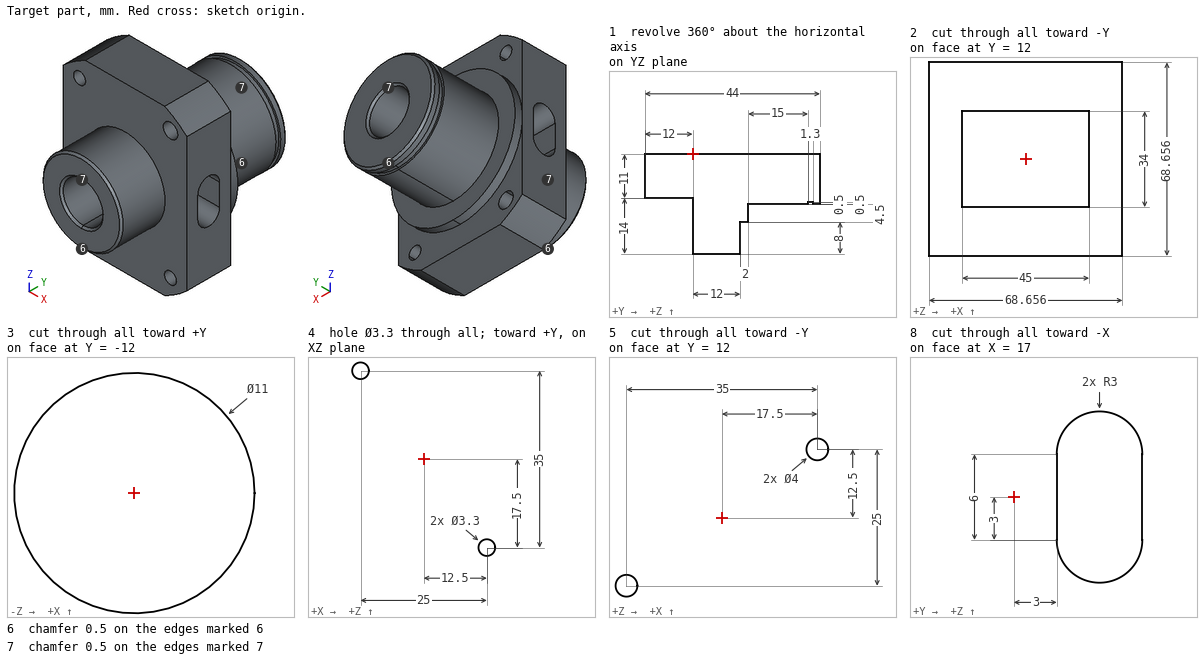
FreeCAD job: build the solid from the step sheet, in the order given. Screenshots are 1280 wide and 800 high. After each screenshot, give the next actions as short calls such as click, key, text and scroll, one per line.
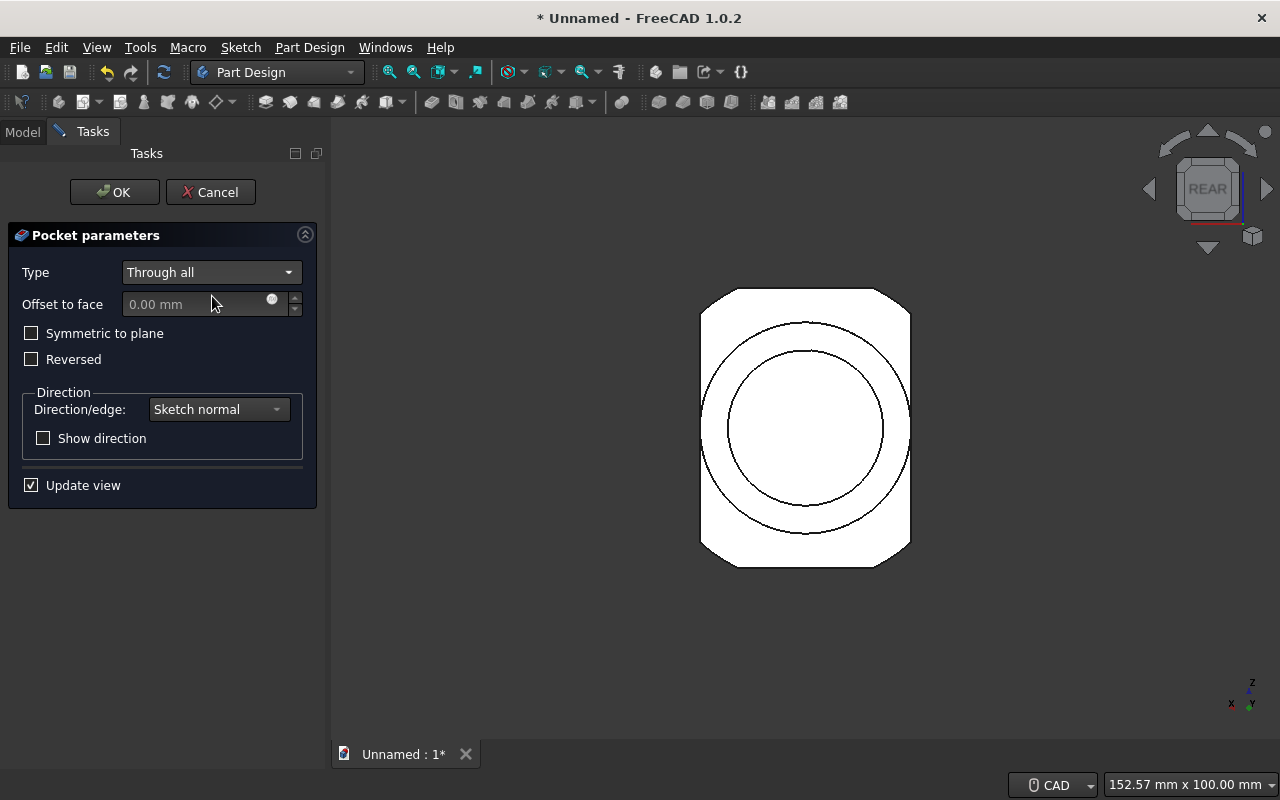
click(115, 192)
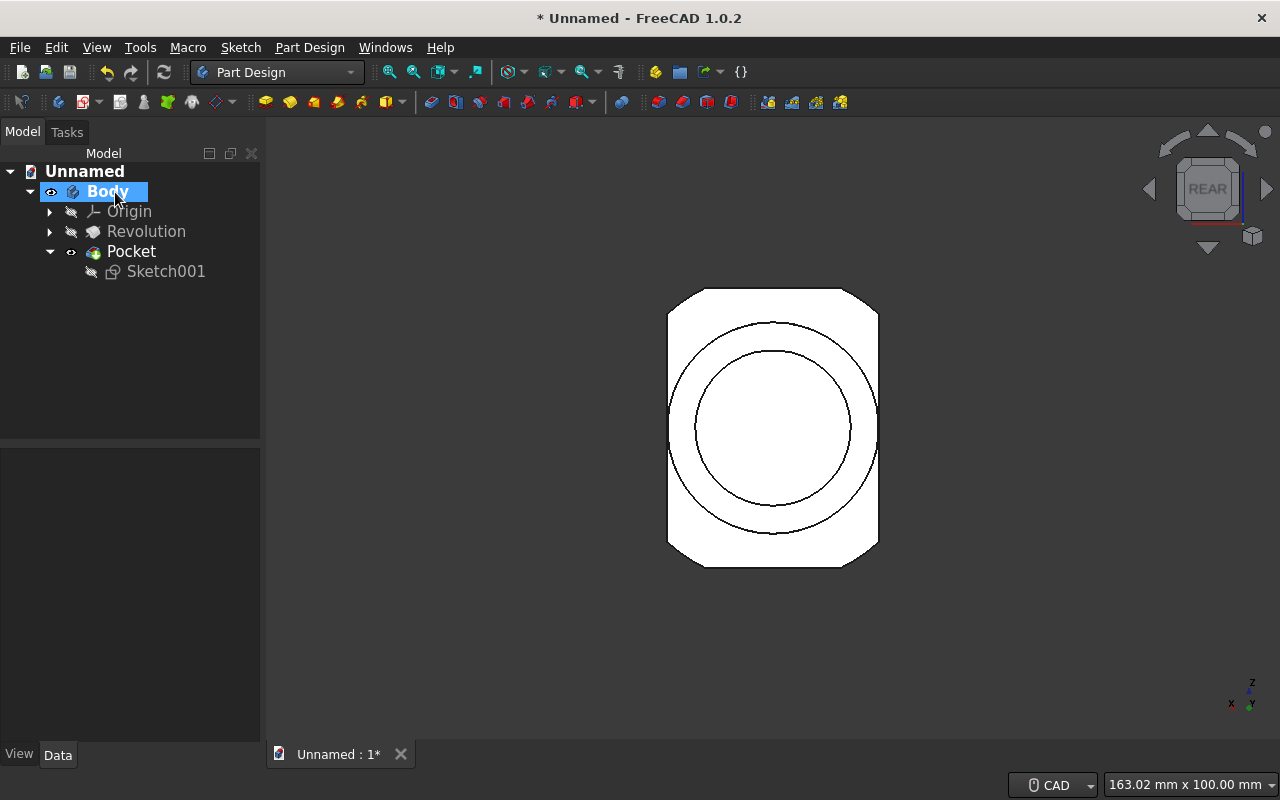
key(0)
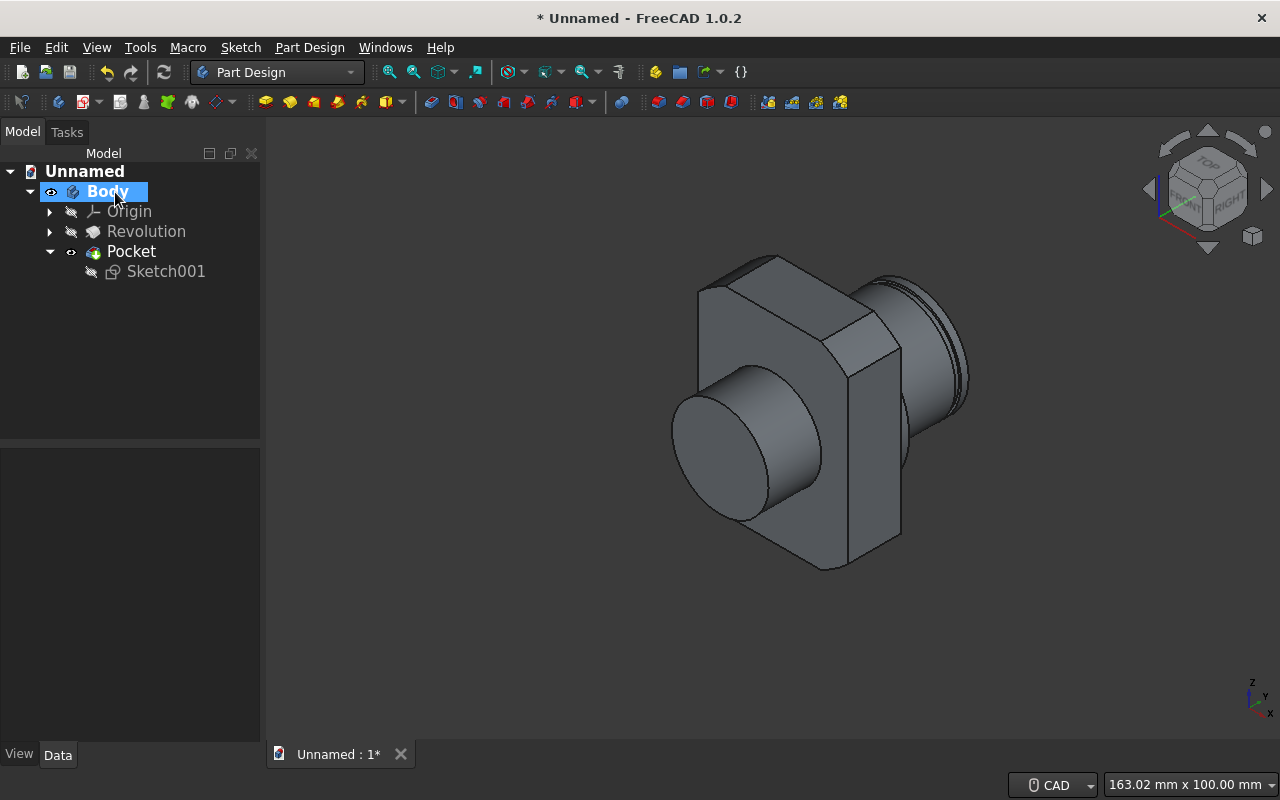
click(720, 457)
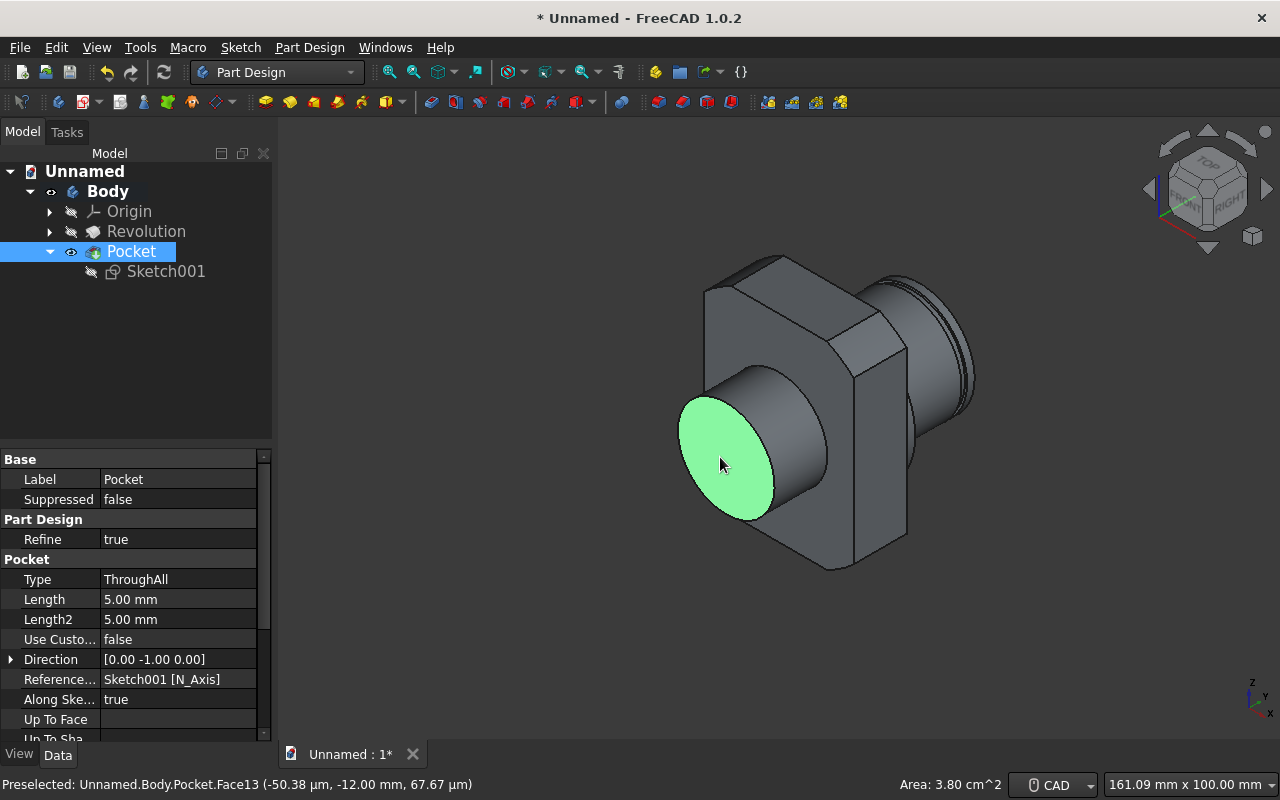
click(84, 102)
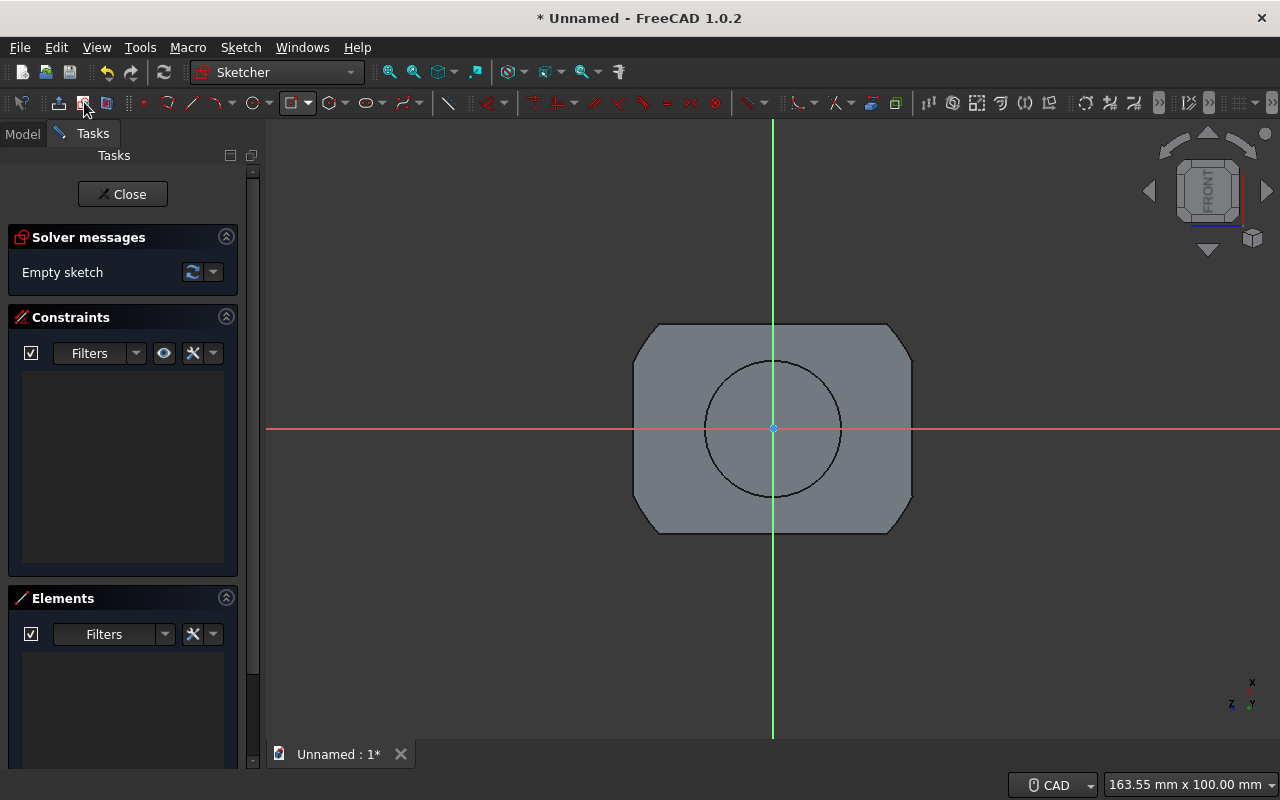
scroll(787, 429, up, 9)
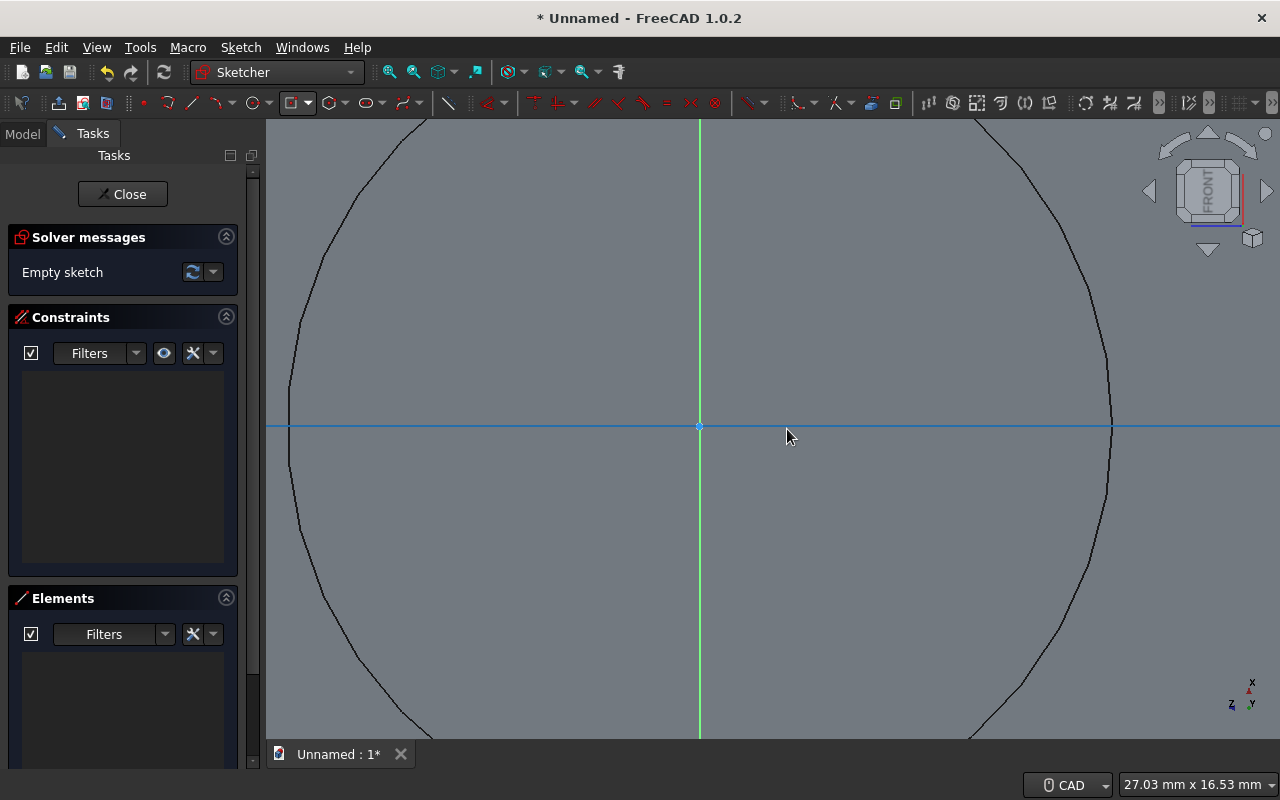
click(254, 104)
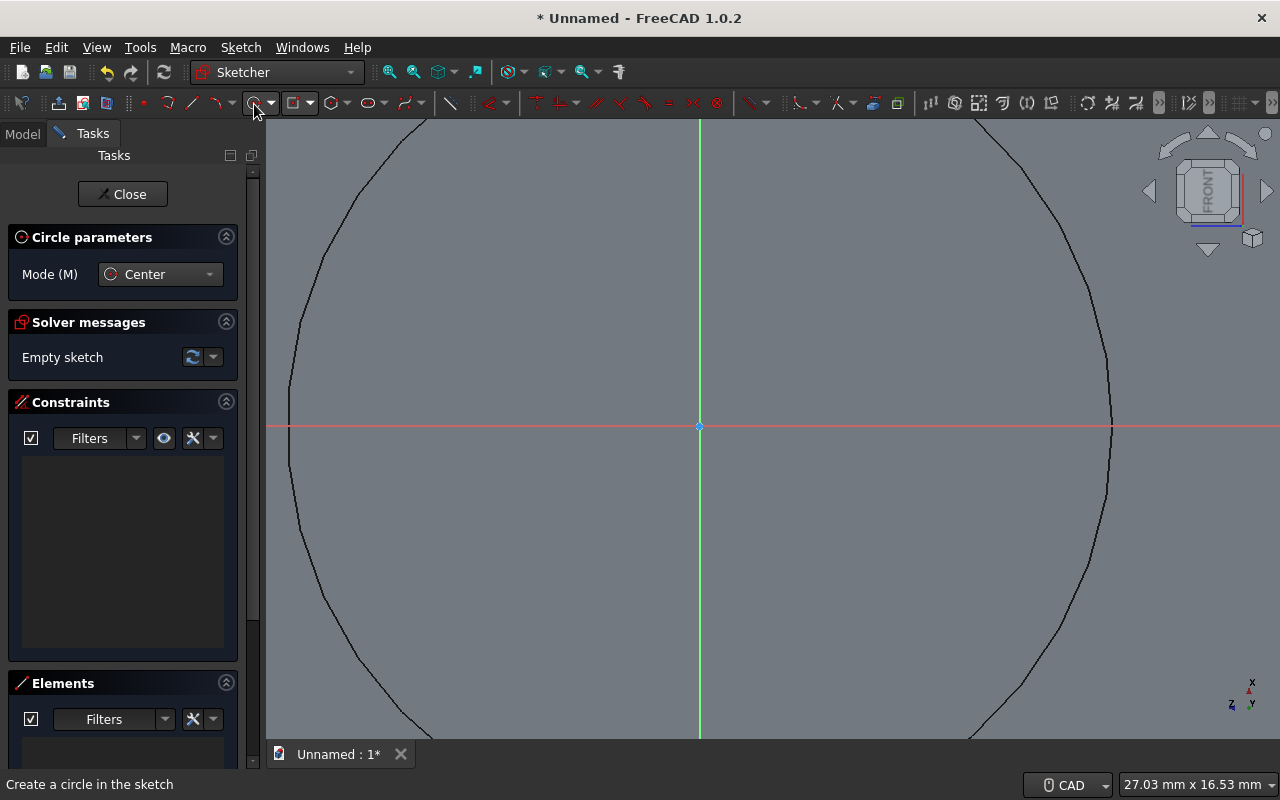
click(700, 426)
move(846, 281)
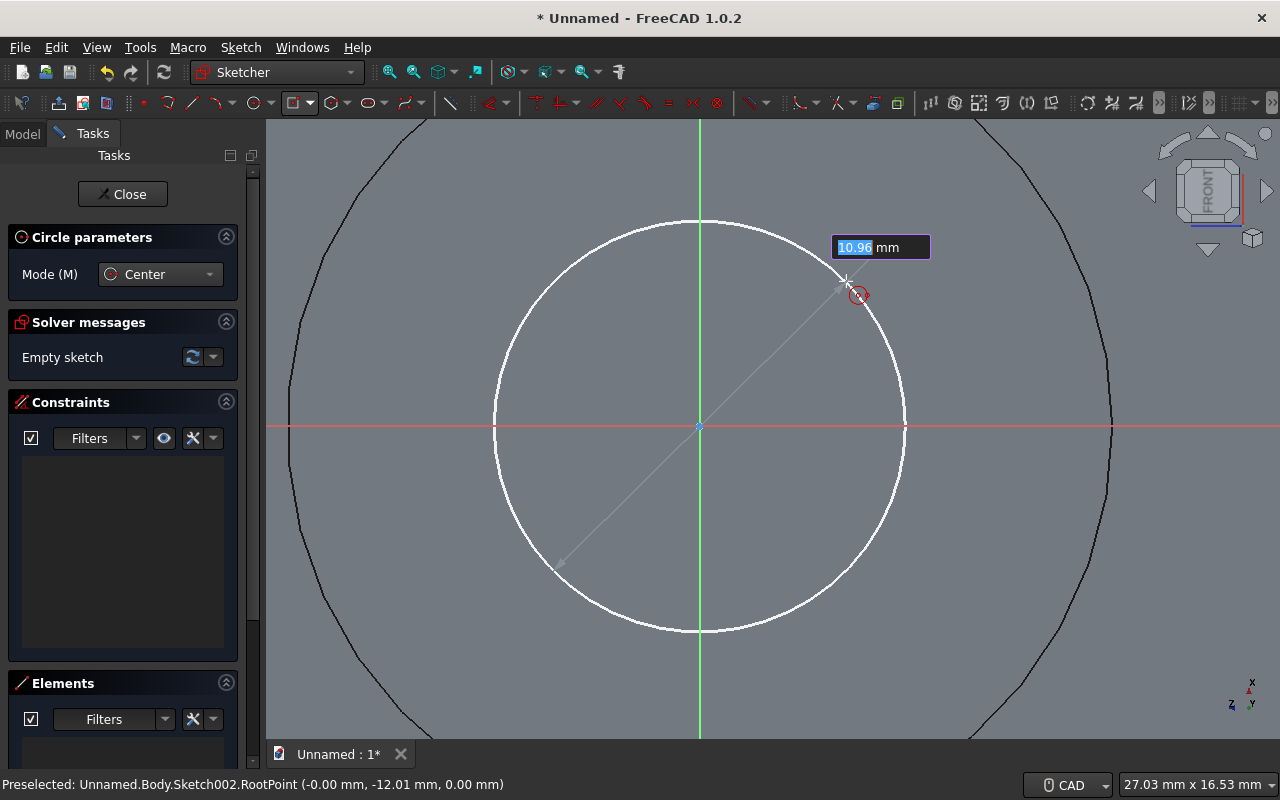
text(11)
key(Return)
key(Escape)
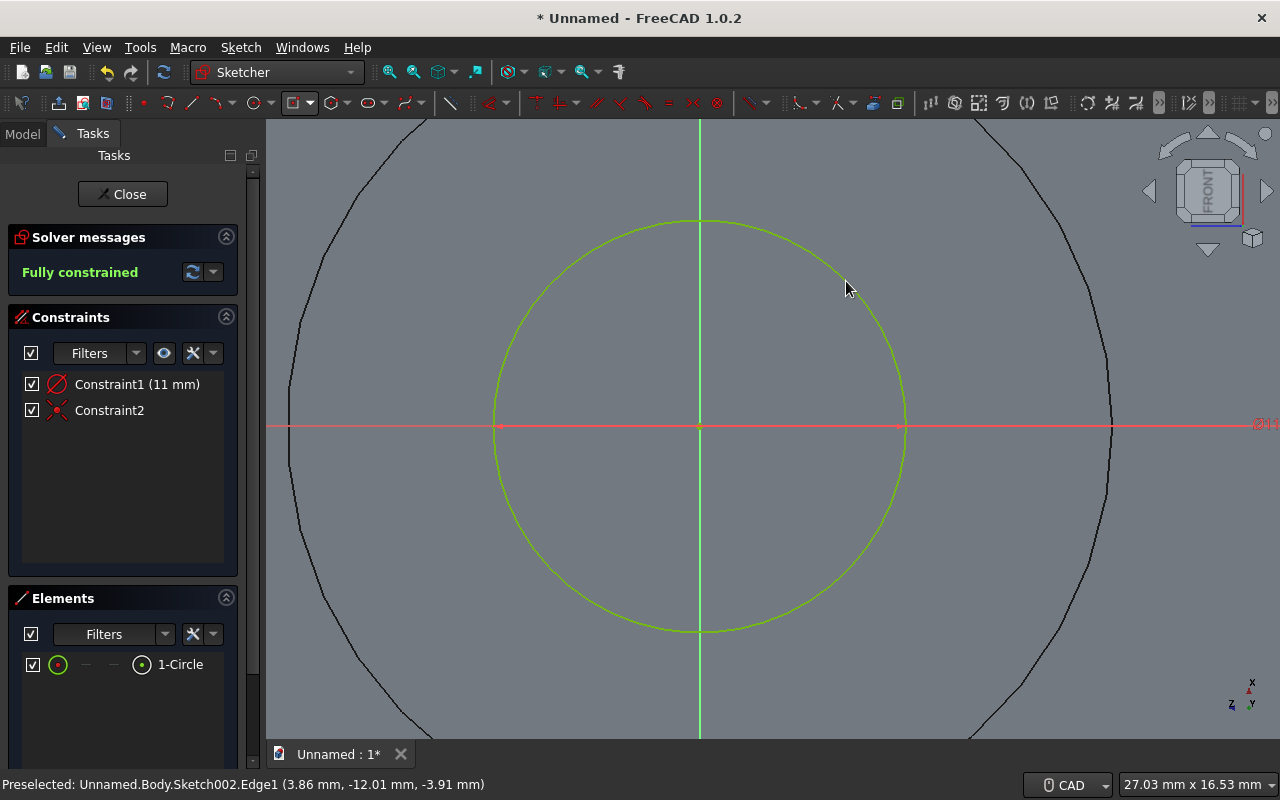
click(123, 194)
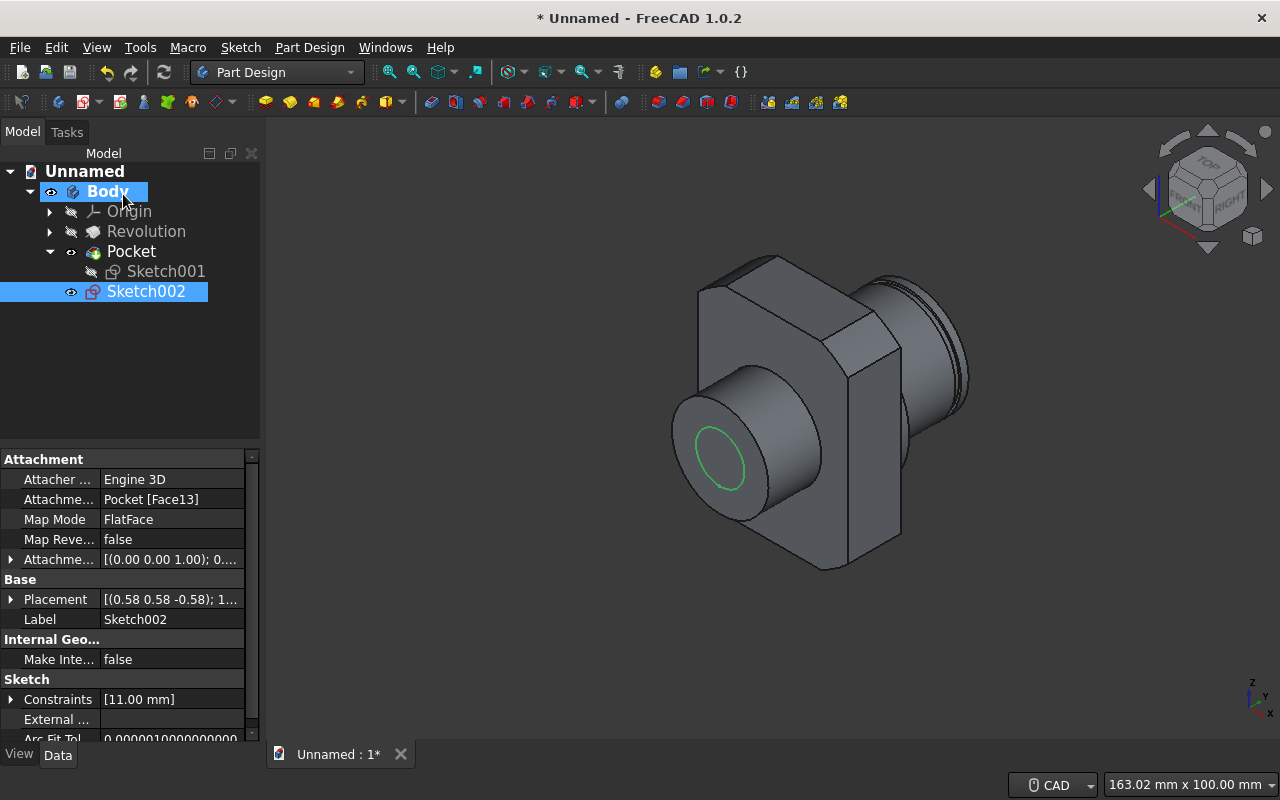
click(432, 102)